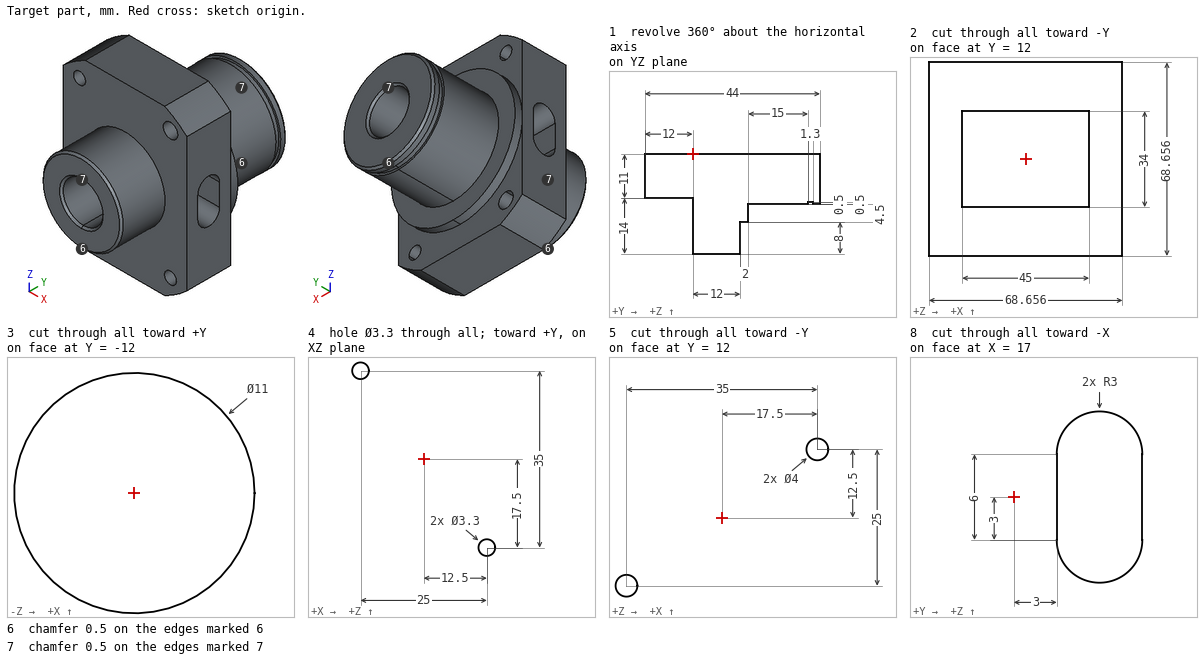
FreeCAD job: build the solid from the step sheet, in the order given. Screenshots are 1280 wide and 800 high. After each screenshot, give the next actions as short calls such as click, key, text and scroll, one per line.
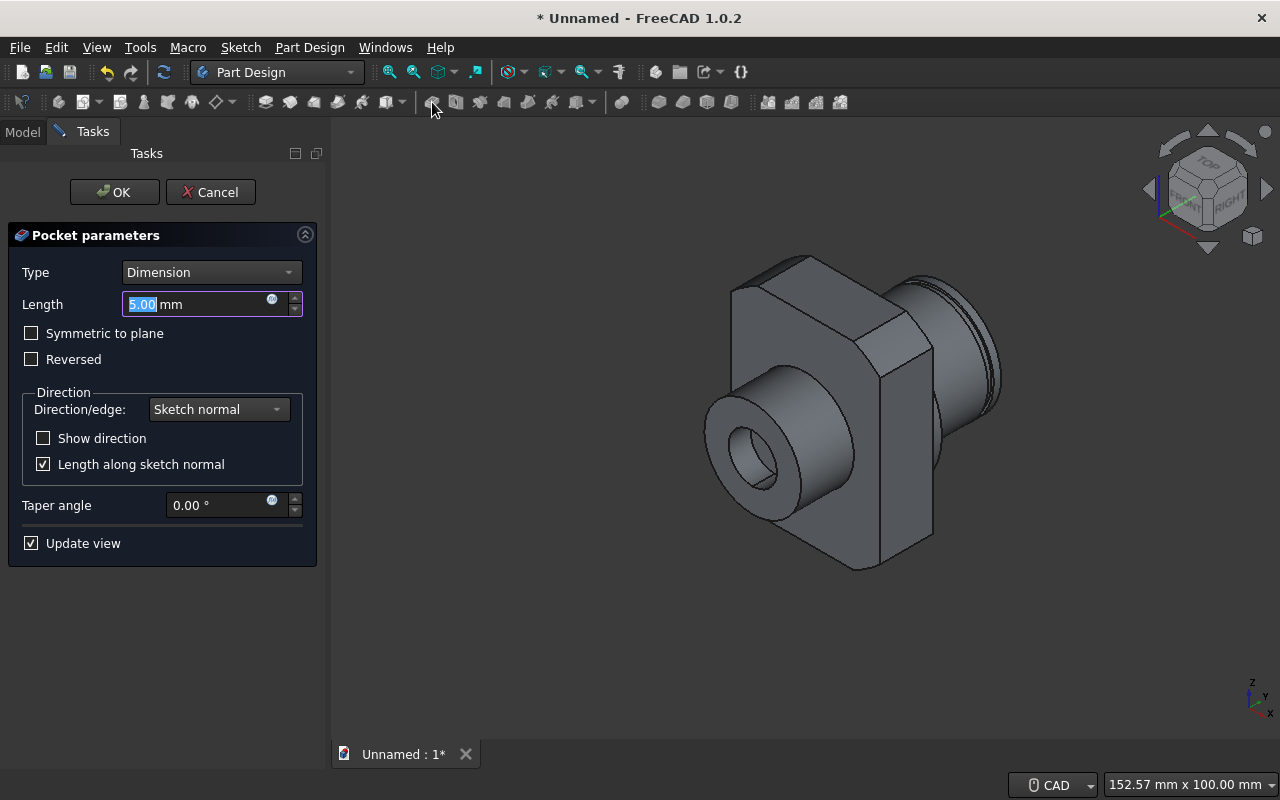
click(212, 272)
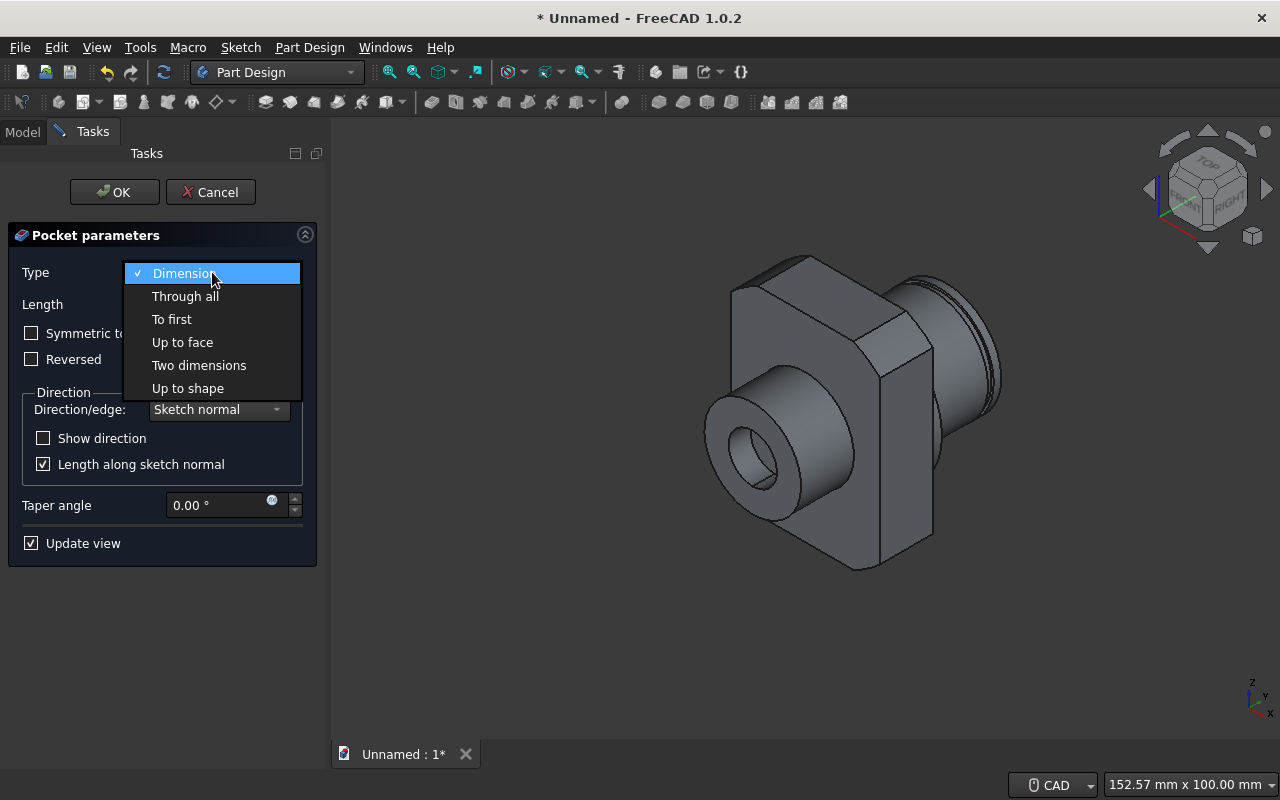
click(212, 296)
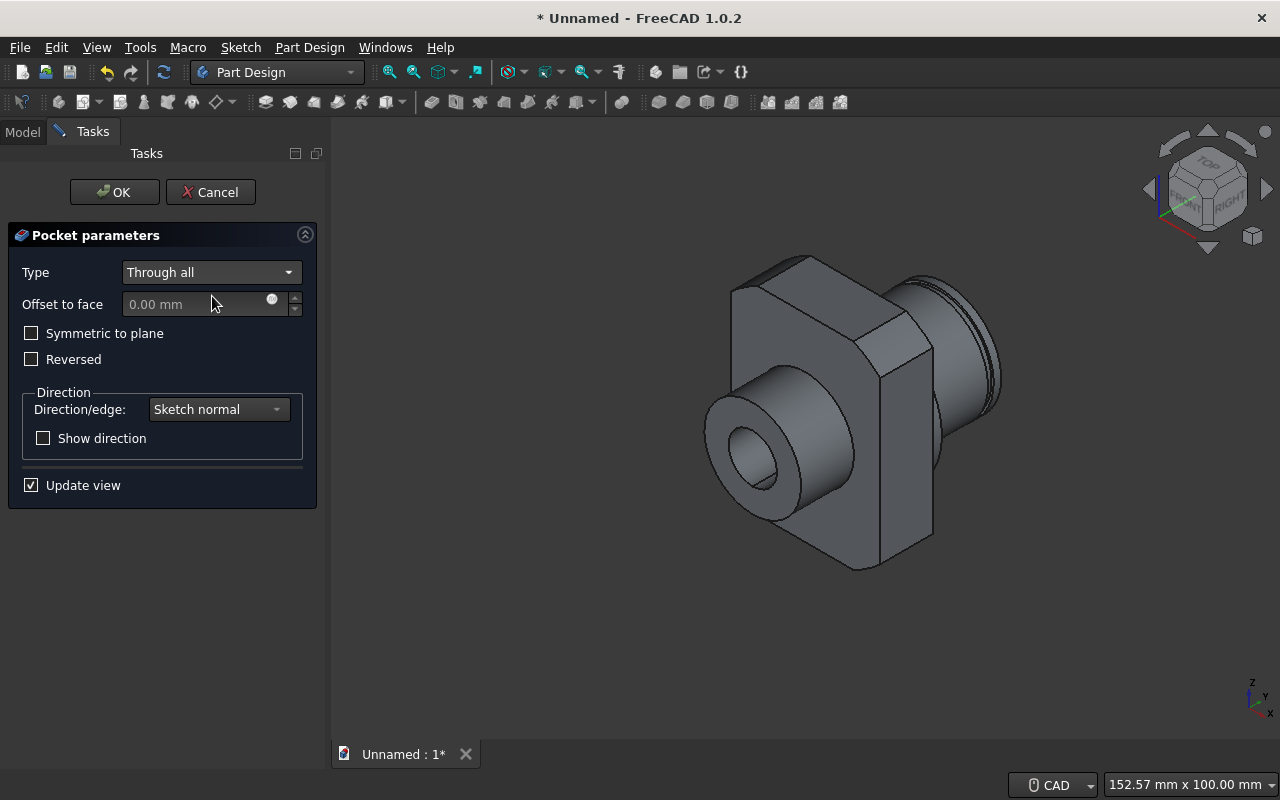
click(115, 192)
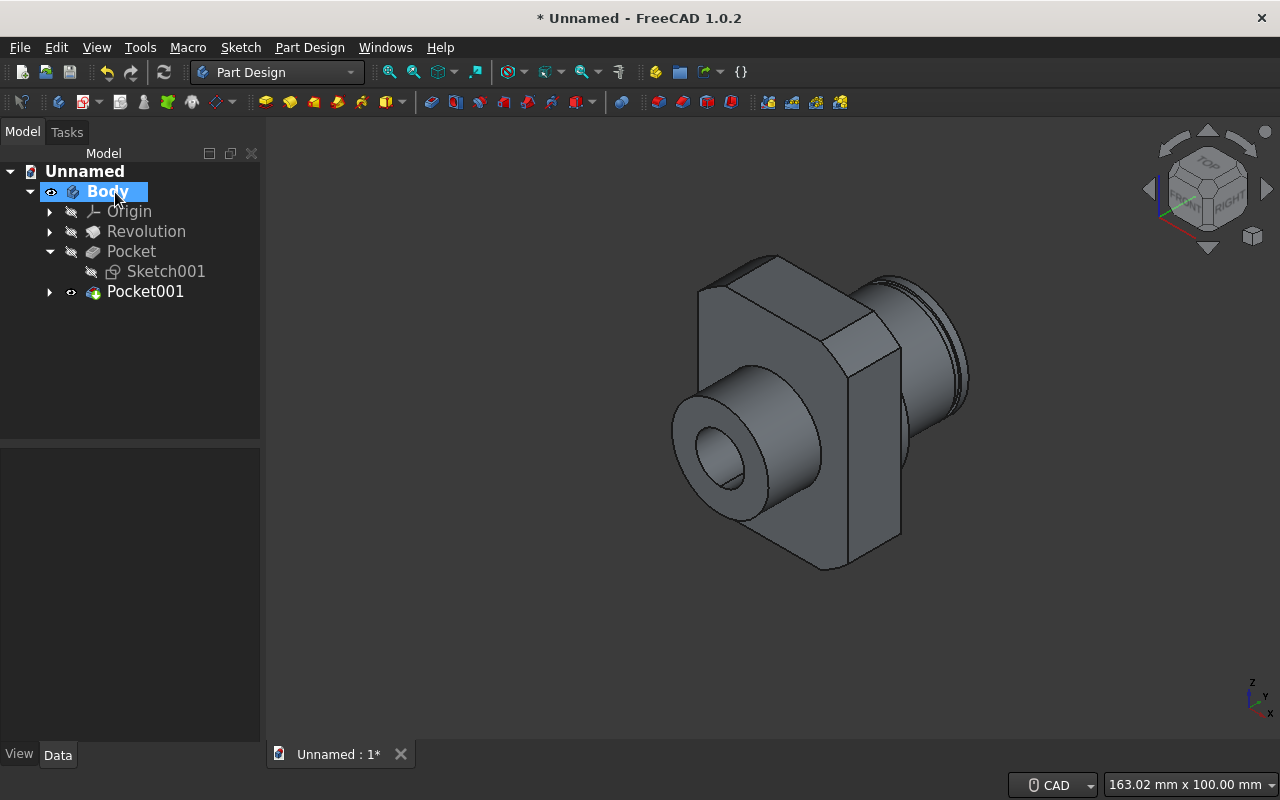
click(84, 102)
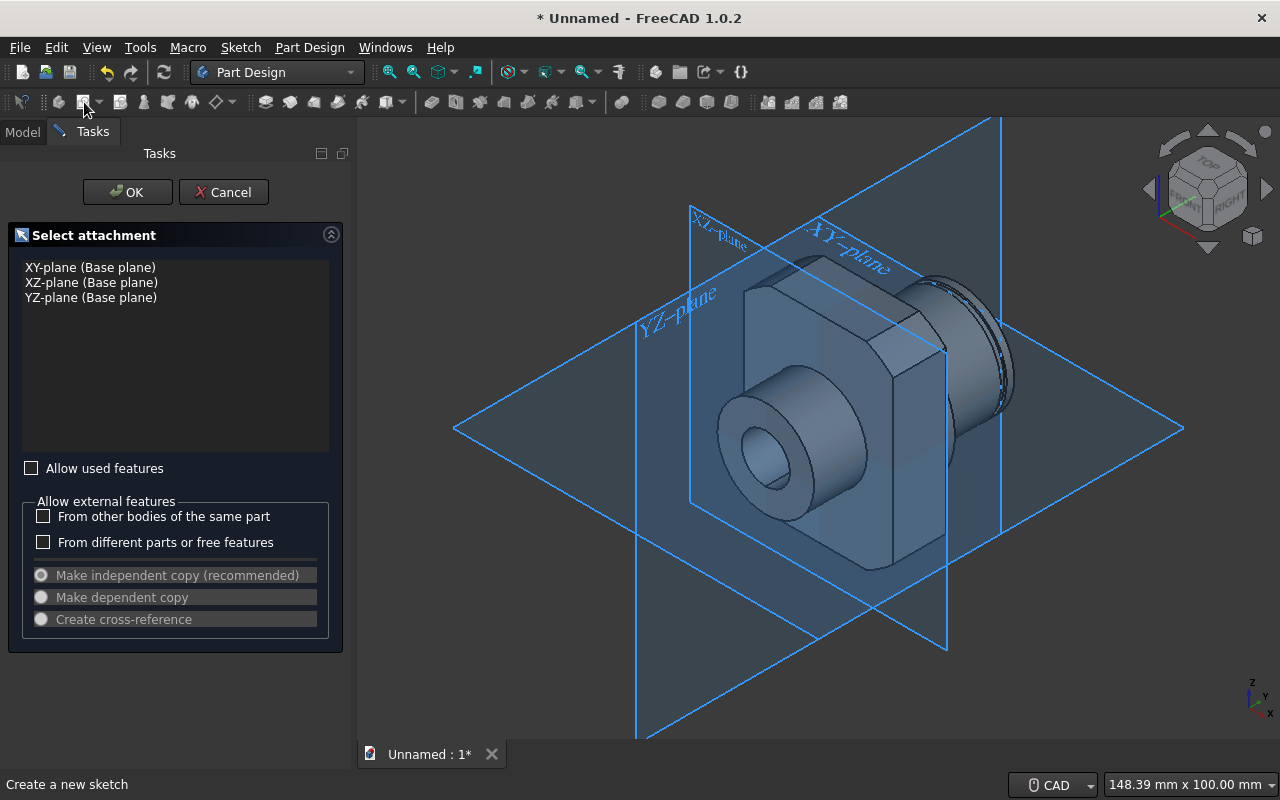
click(82, 282)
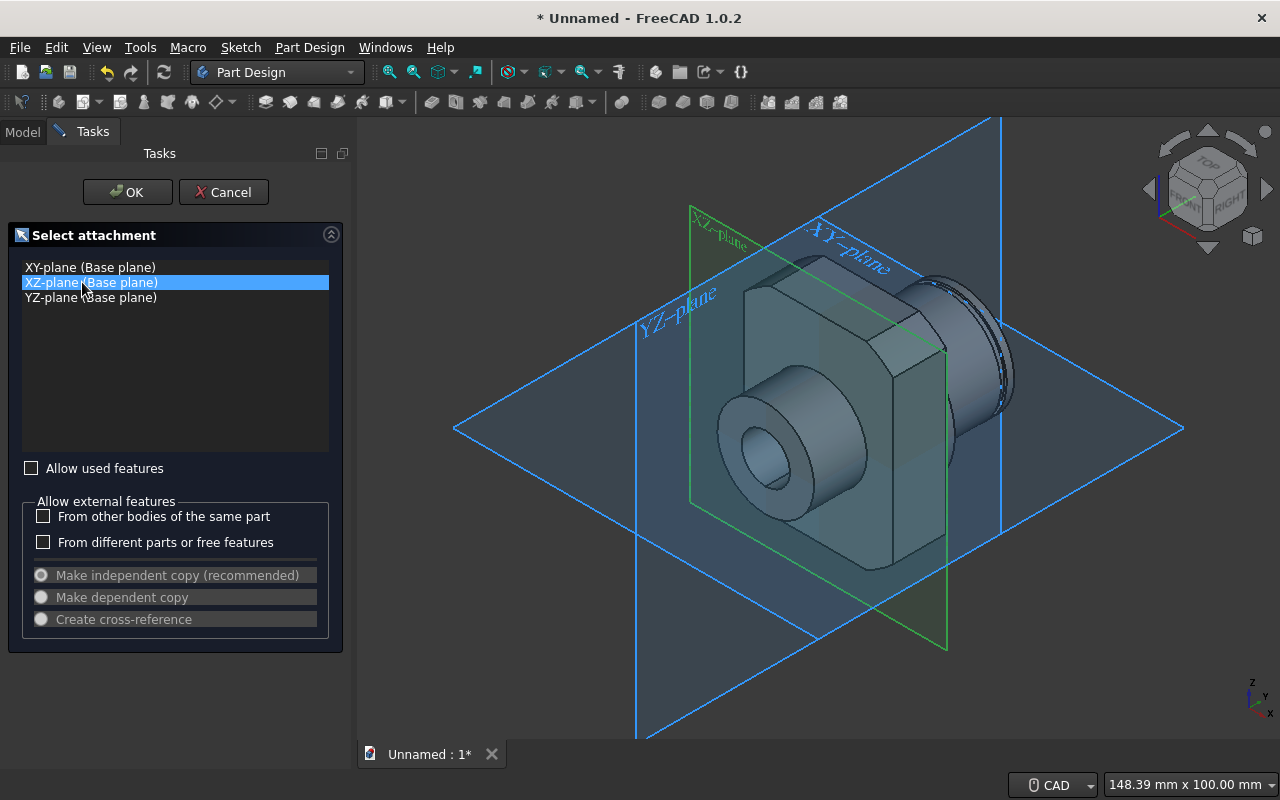
click(128, 192)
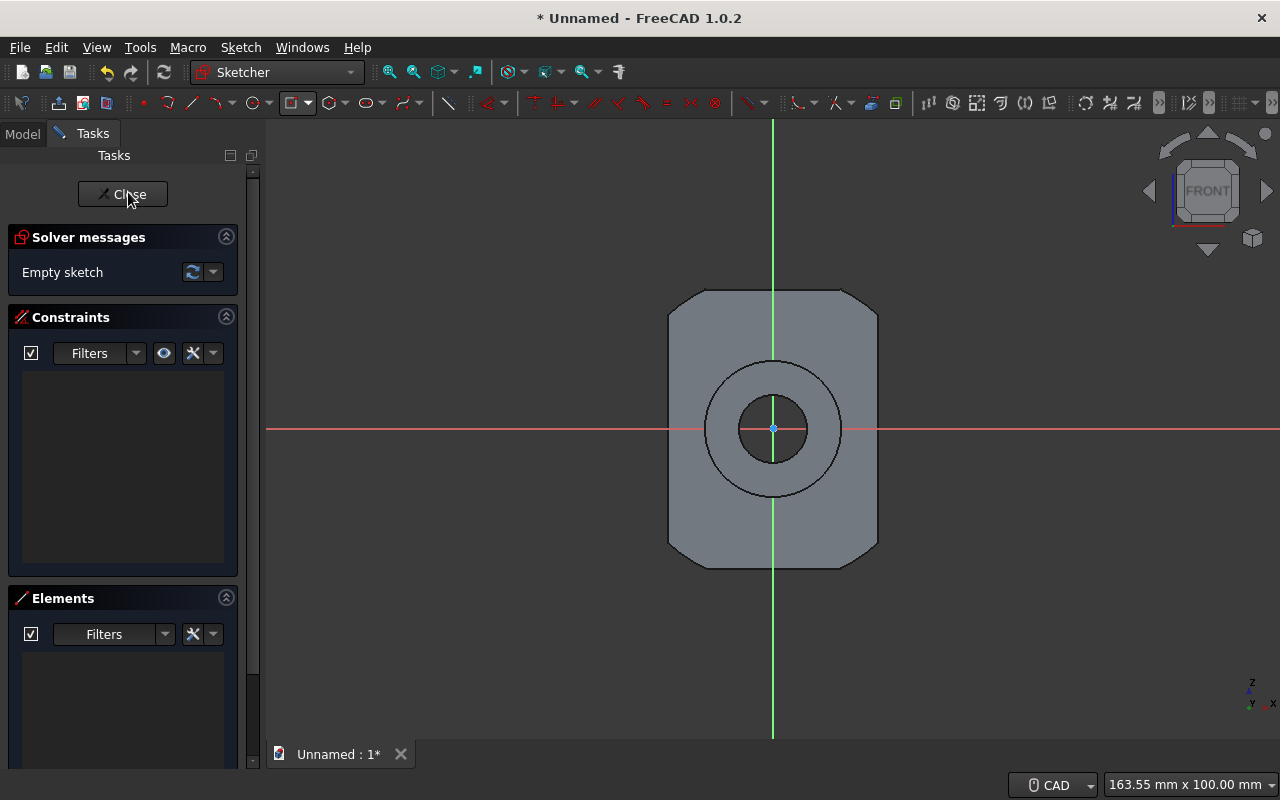
click(108, 104)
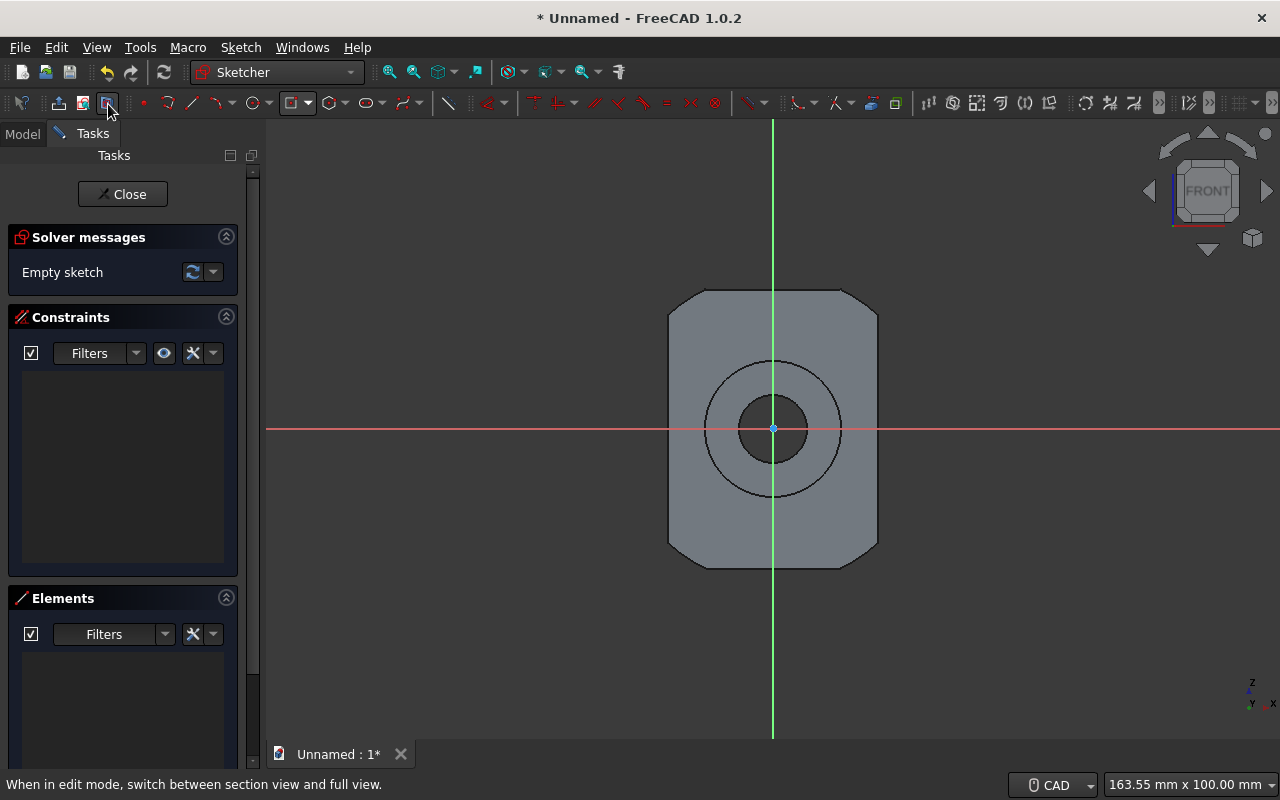
scroll(856, 429, up, 3)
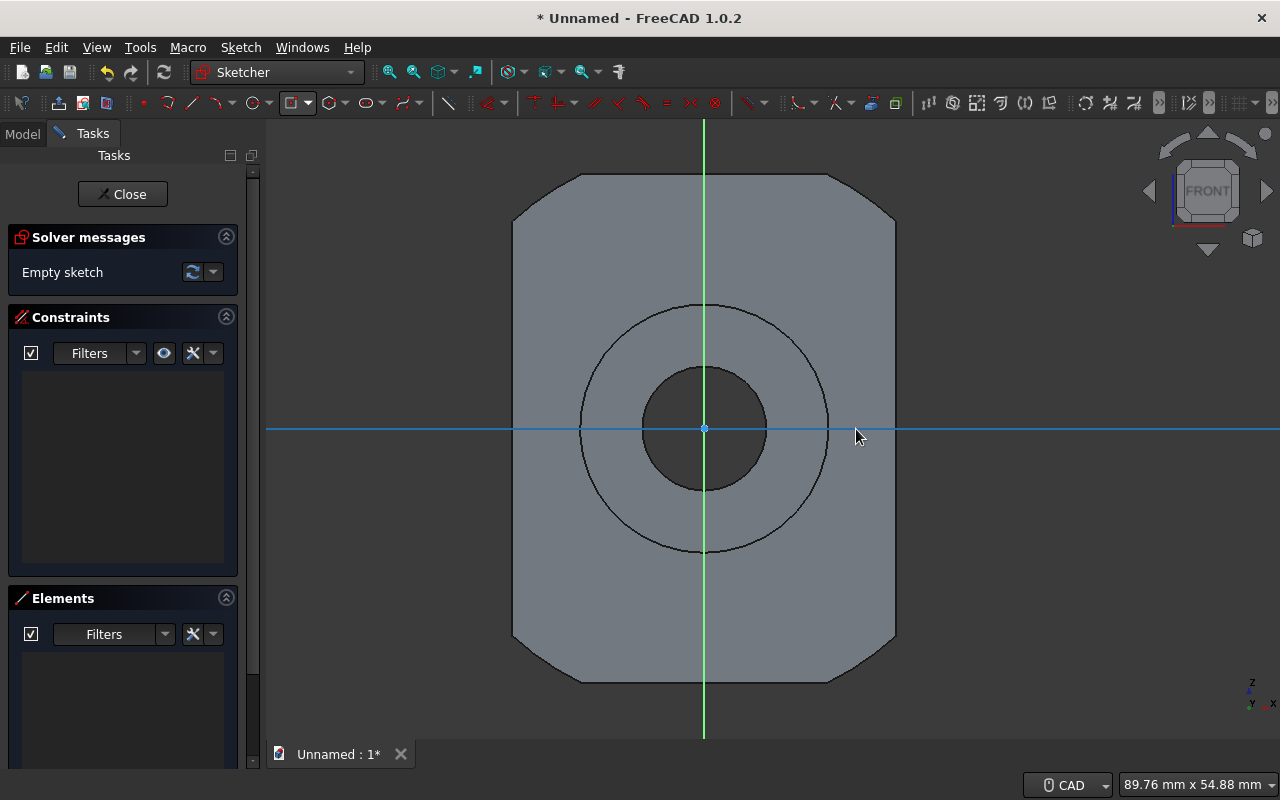
click(254, 104)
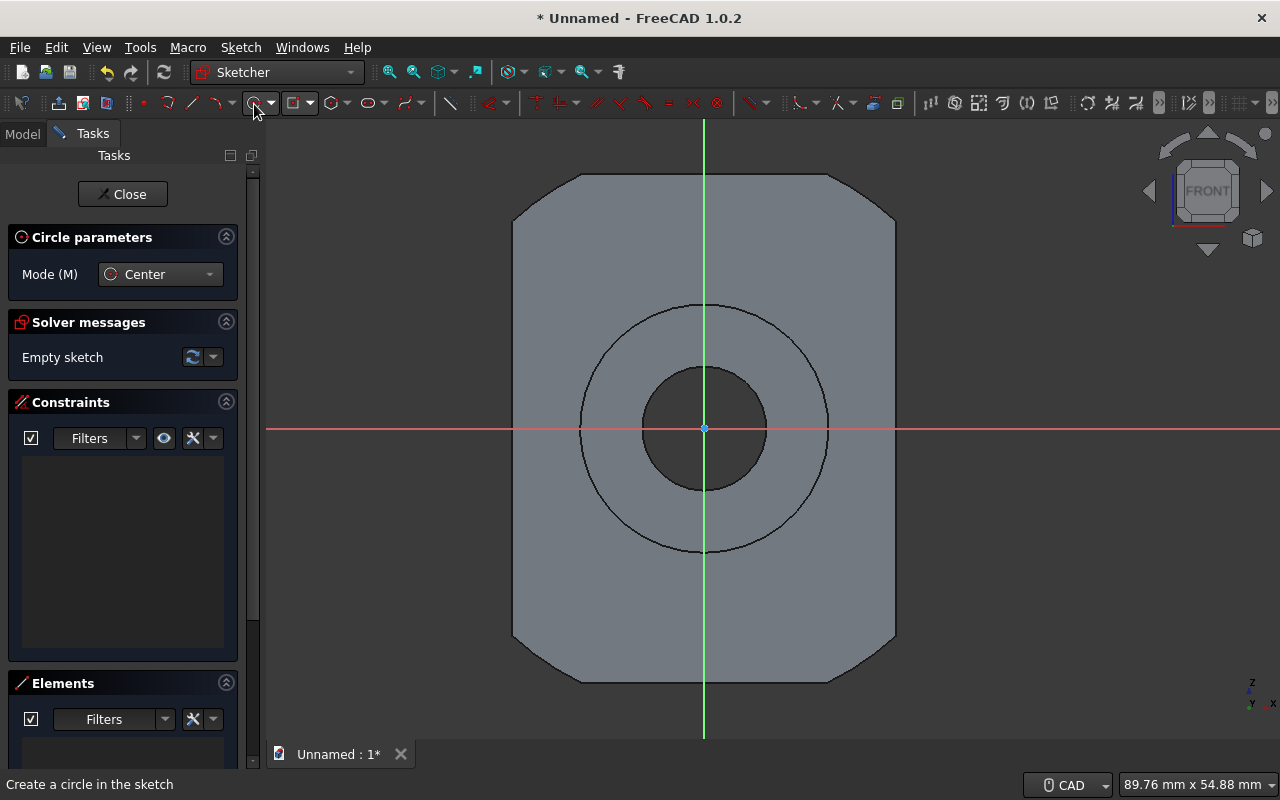
click(845, 626)
move(859, 613)